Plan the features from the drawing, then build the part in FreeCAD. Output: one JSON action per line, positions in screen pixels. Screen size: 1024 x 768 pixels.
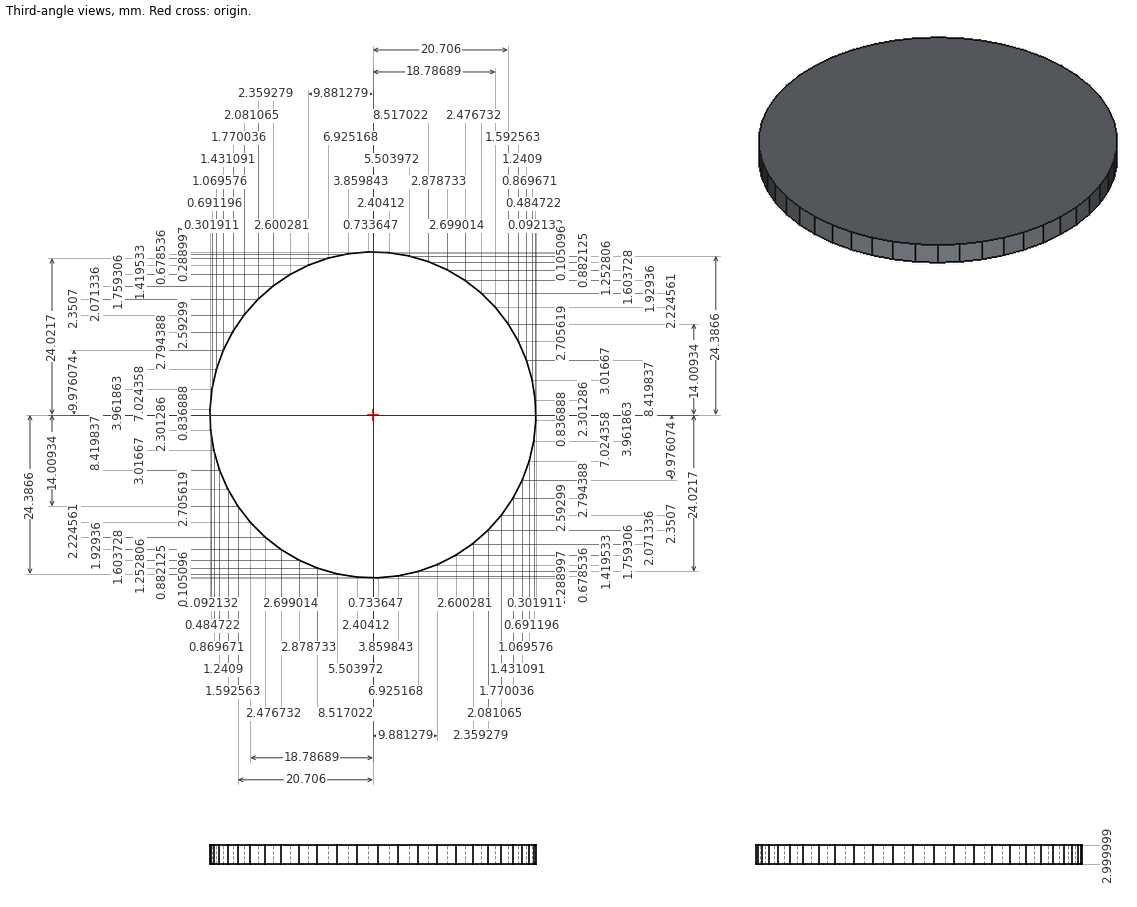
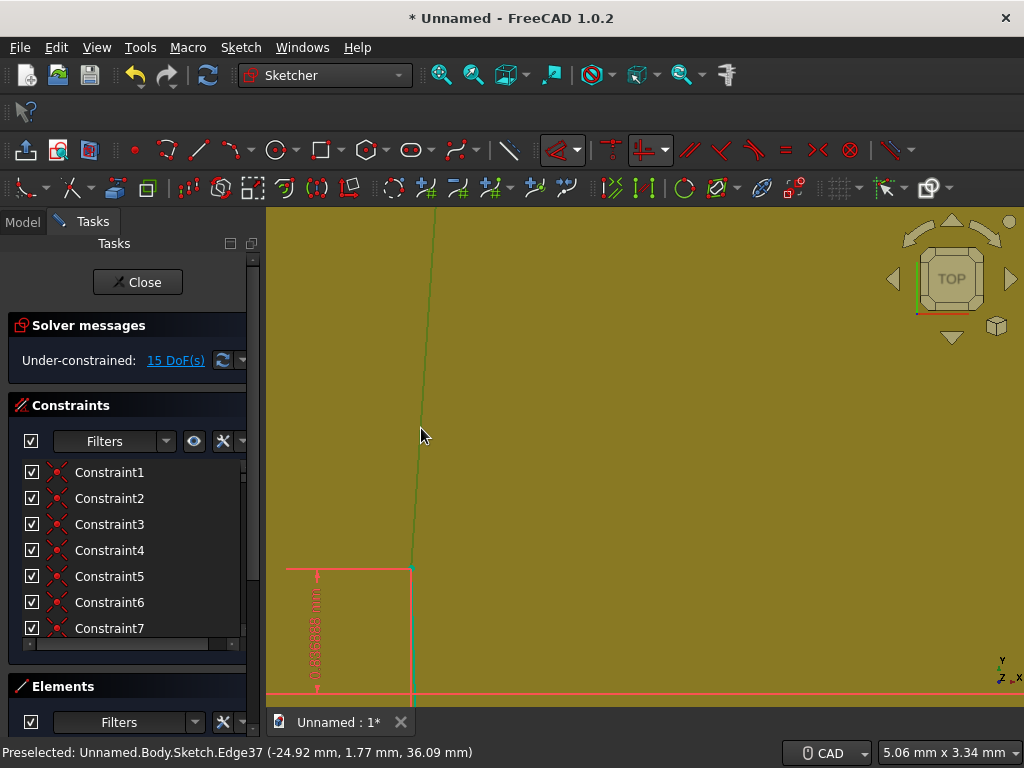
{"action": "left_click", "coordinate": [580, 150]}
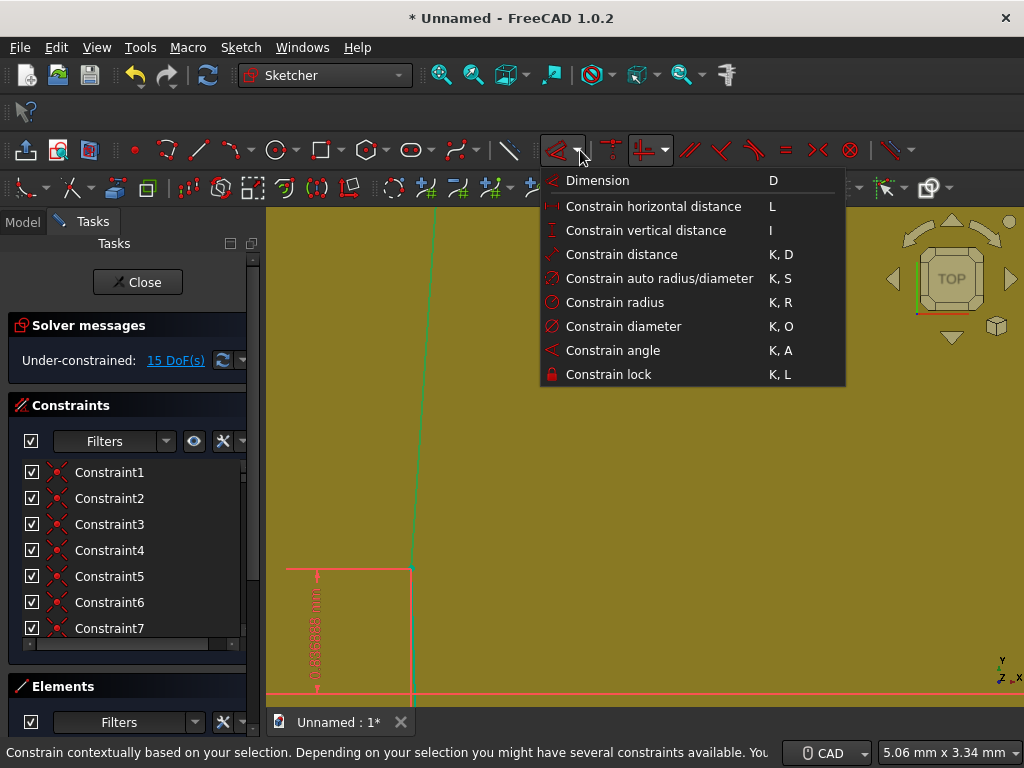
{"action": "left_click", "coordinate": [693, 206]}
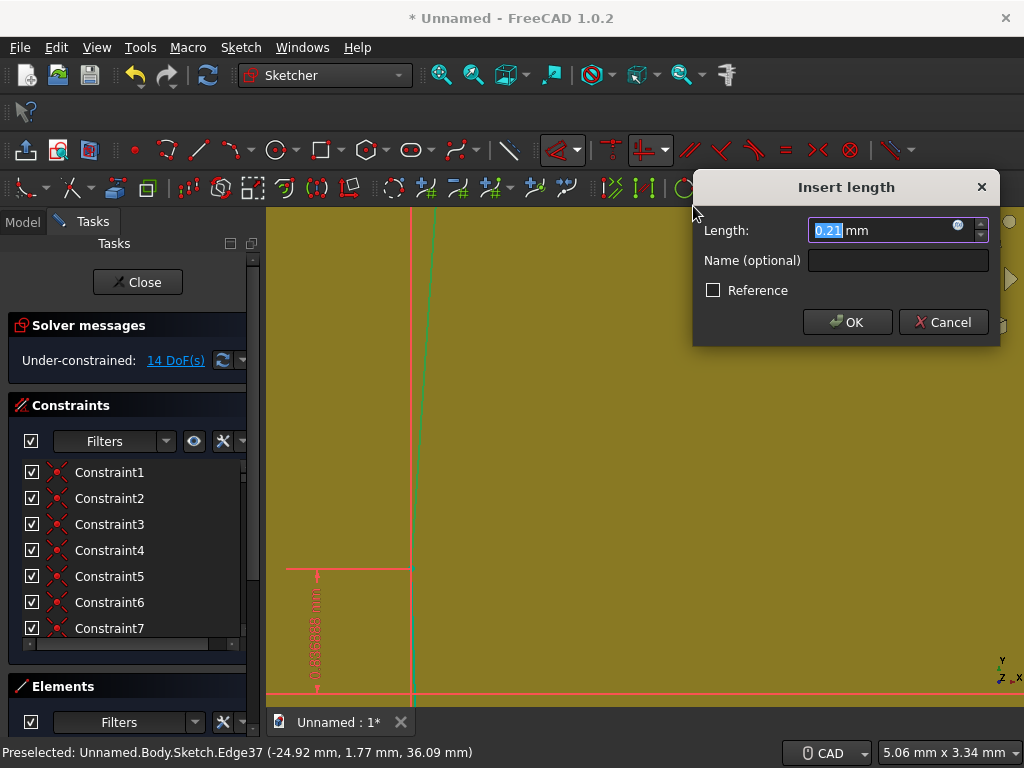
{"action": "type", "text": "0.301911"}
{"action": "key", "text": "Return"}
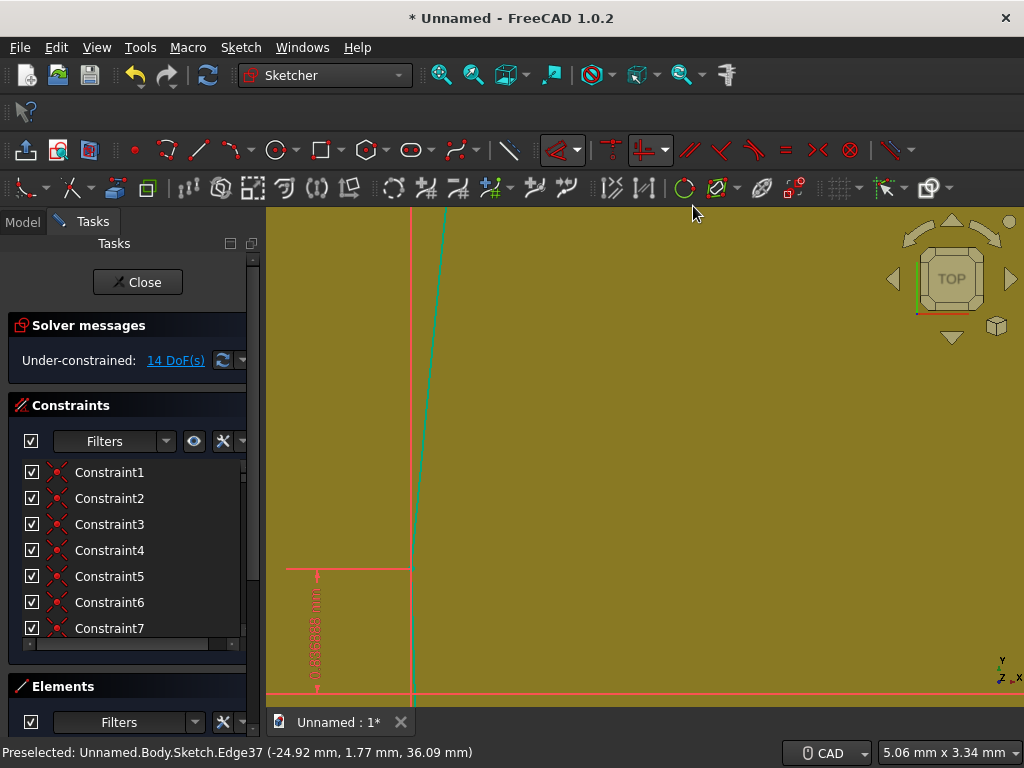
{"action": "scroll", "coordinate": [389, 445], "scroll_direction": "down", "scroll_amount": 15}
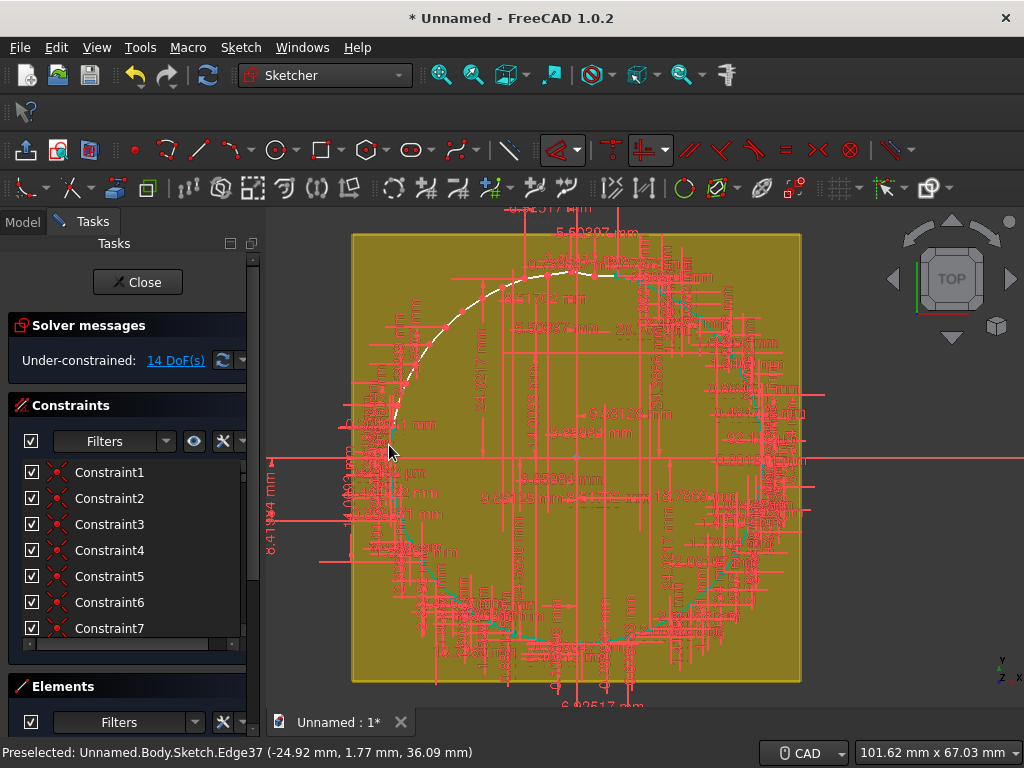
{"action": "scroll", "coordinate": [394, 421], "scroll_direction": "up", "scroll_amount": 11}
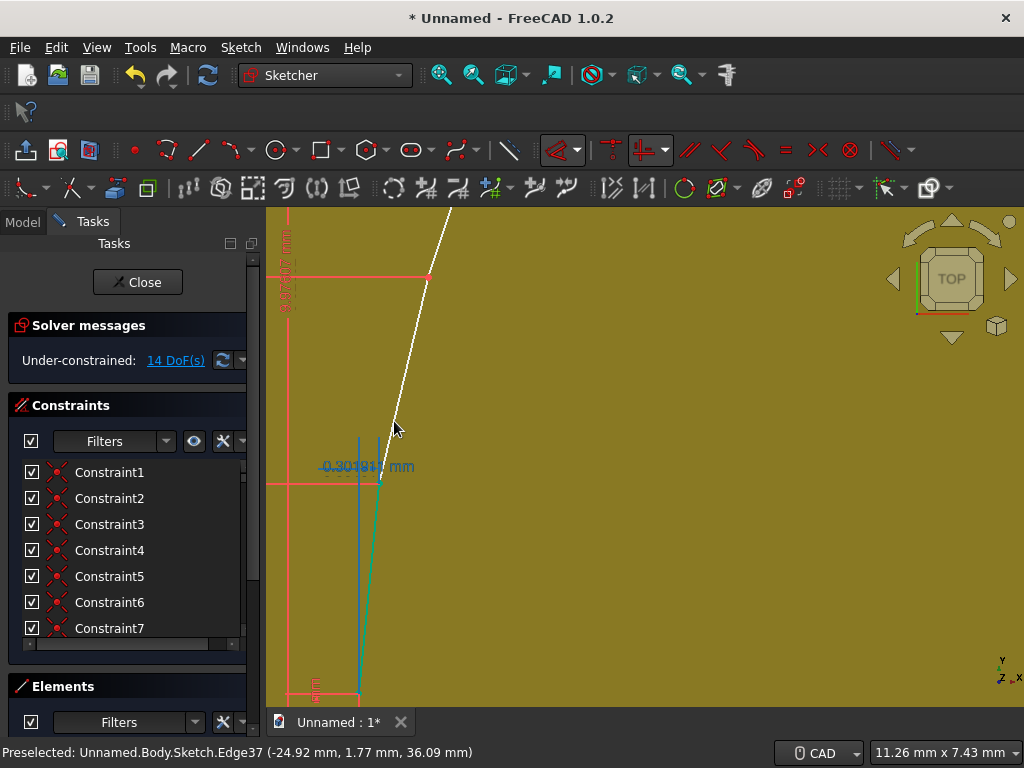
{"action": "left_click", "coordinate": [394, 422]}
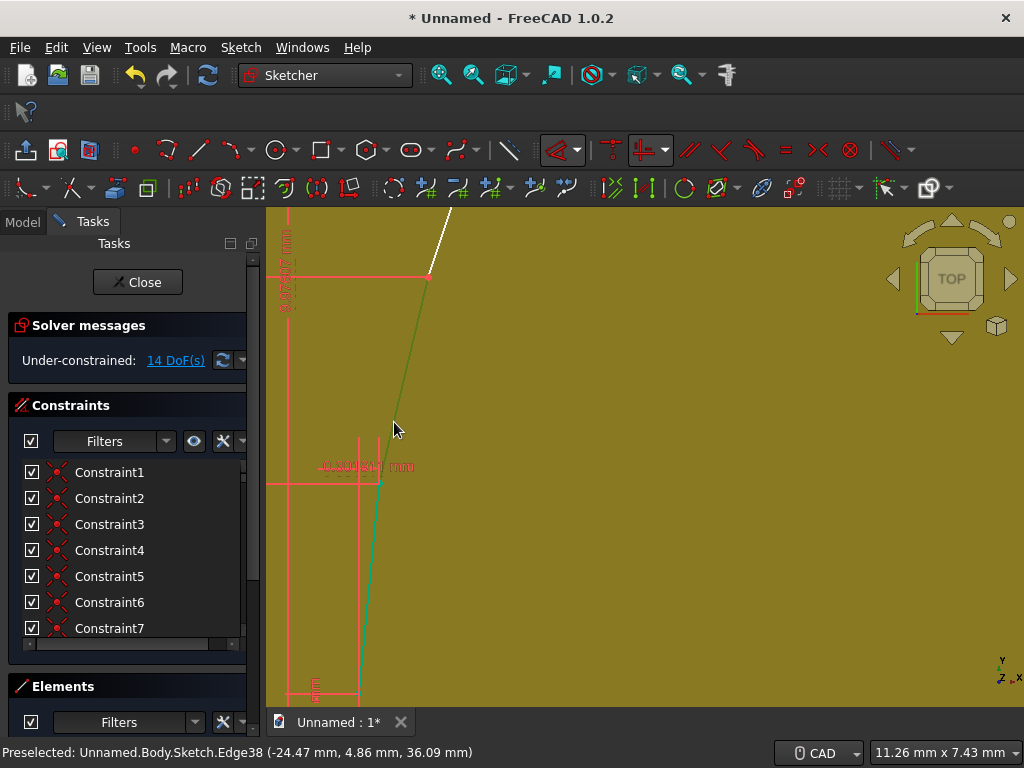
{"action": "left_click", "coordinate": [580, 150]}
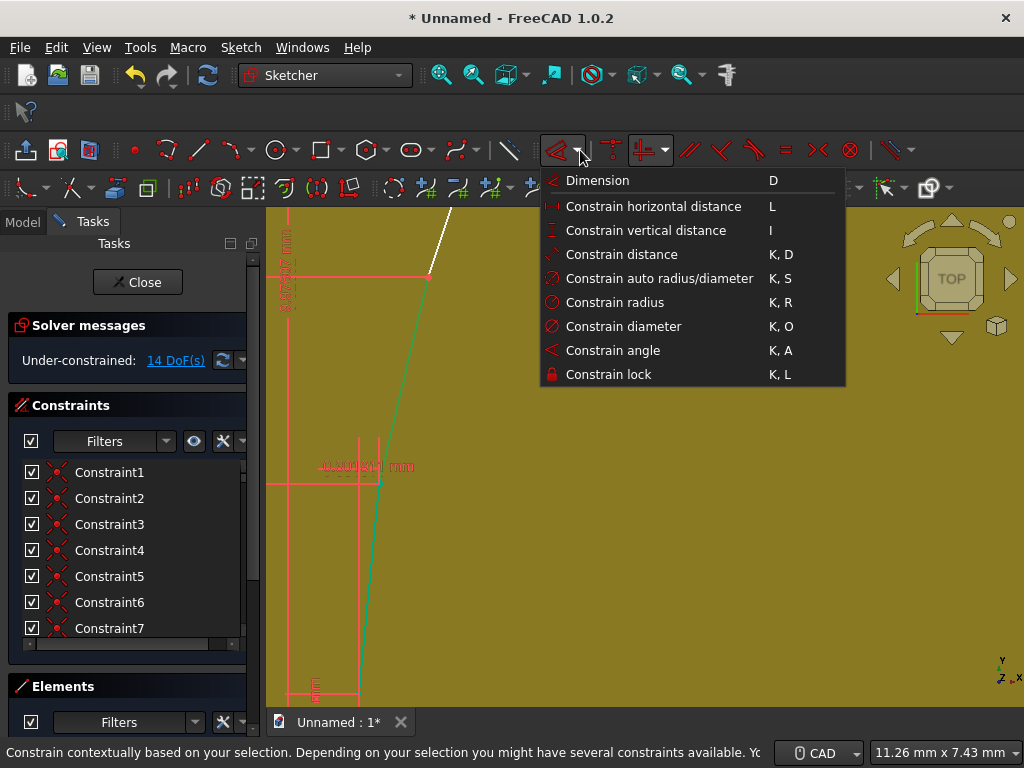
{"action": "left_click", "coordinate": [693, 206]}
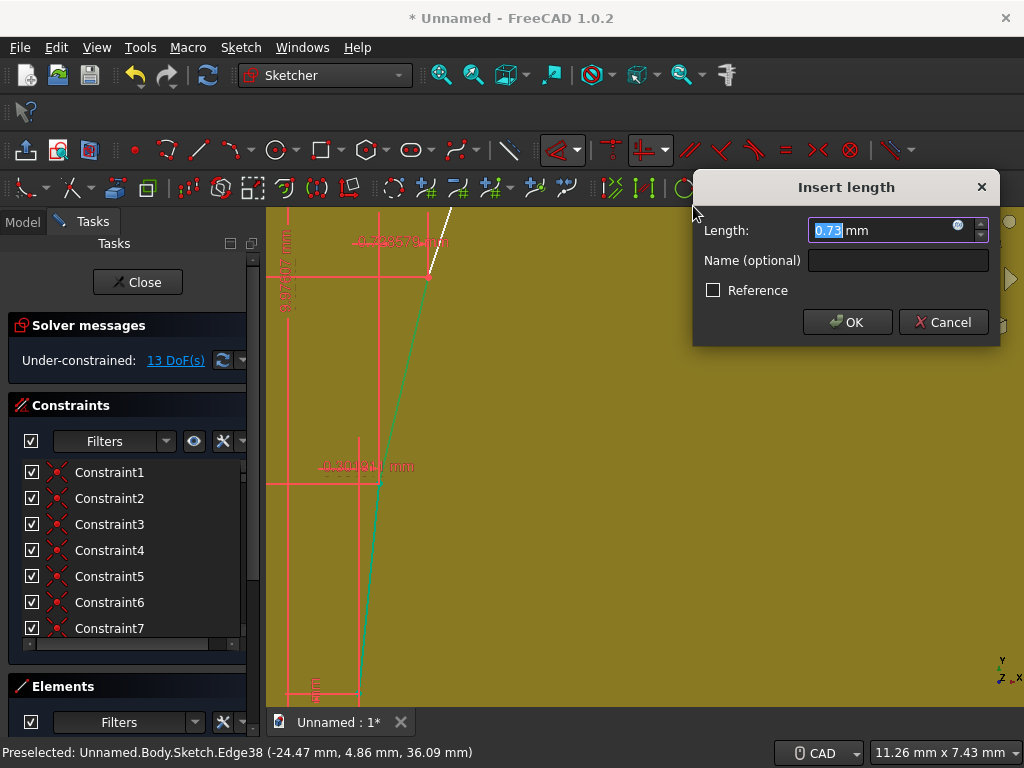
{"action": "type", "text": "0.691196"}
{"action": "key", "text": "Return"}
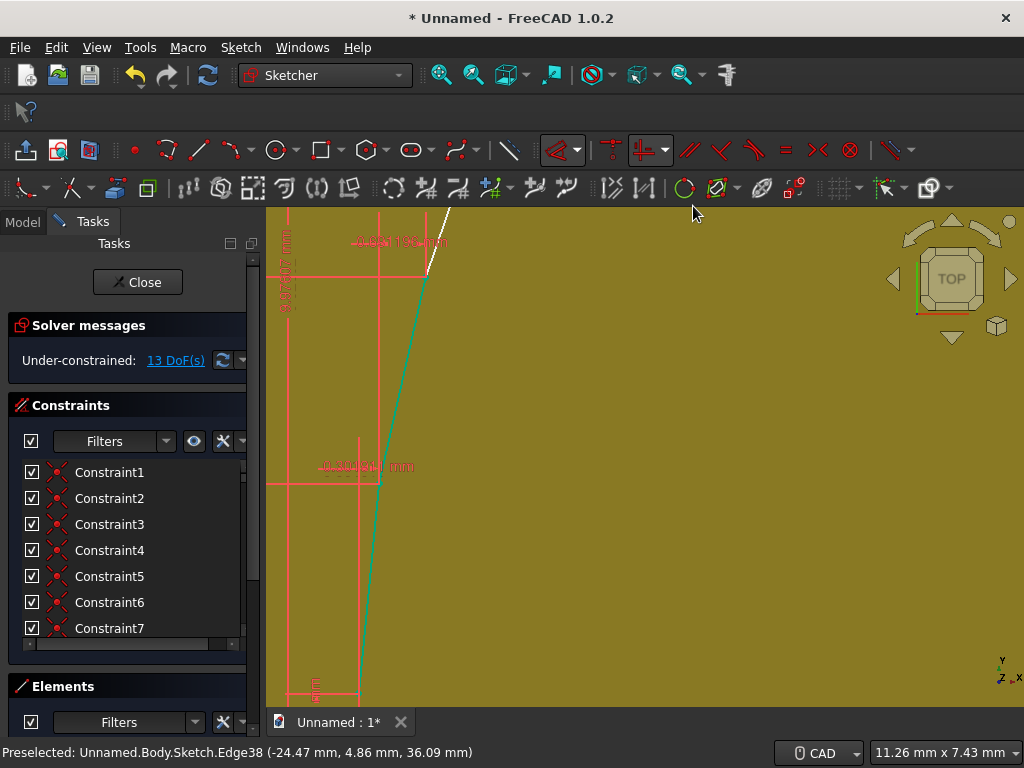
{"action": "scroll", "coordinate": [439, 238], "scroll_direction": "up", "scroll_amount": 4}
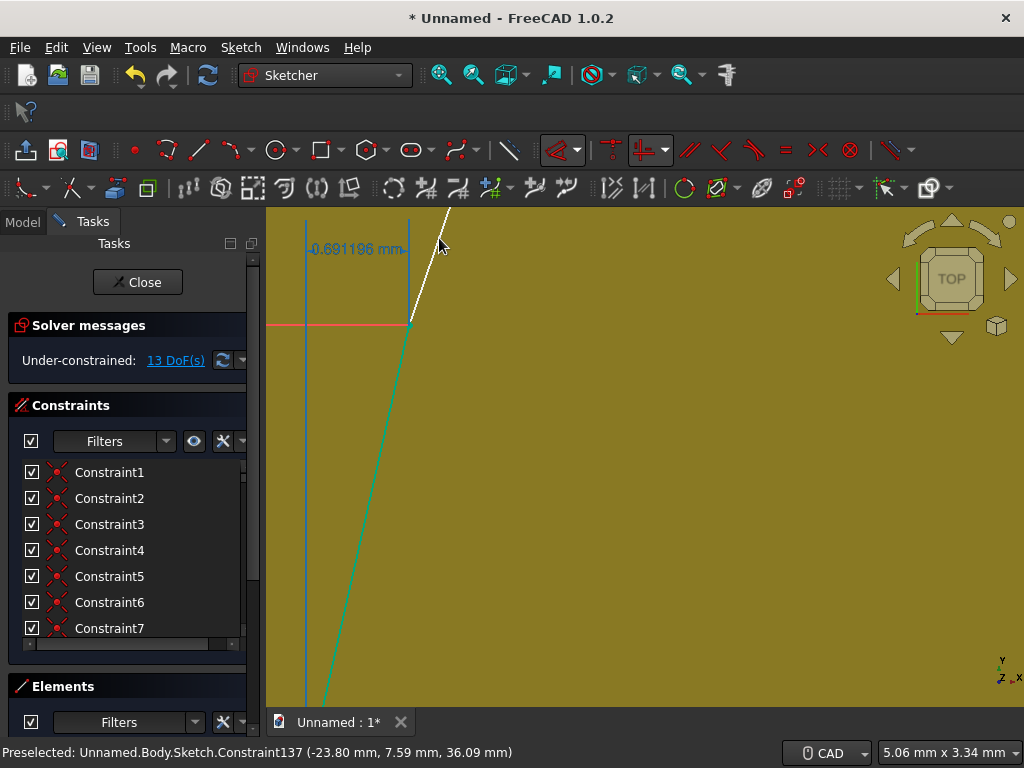
{"action": "left_click", "coordinate": [440, 237]}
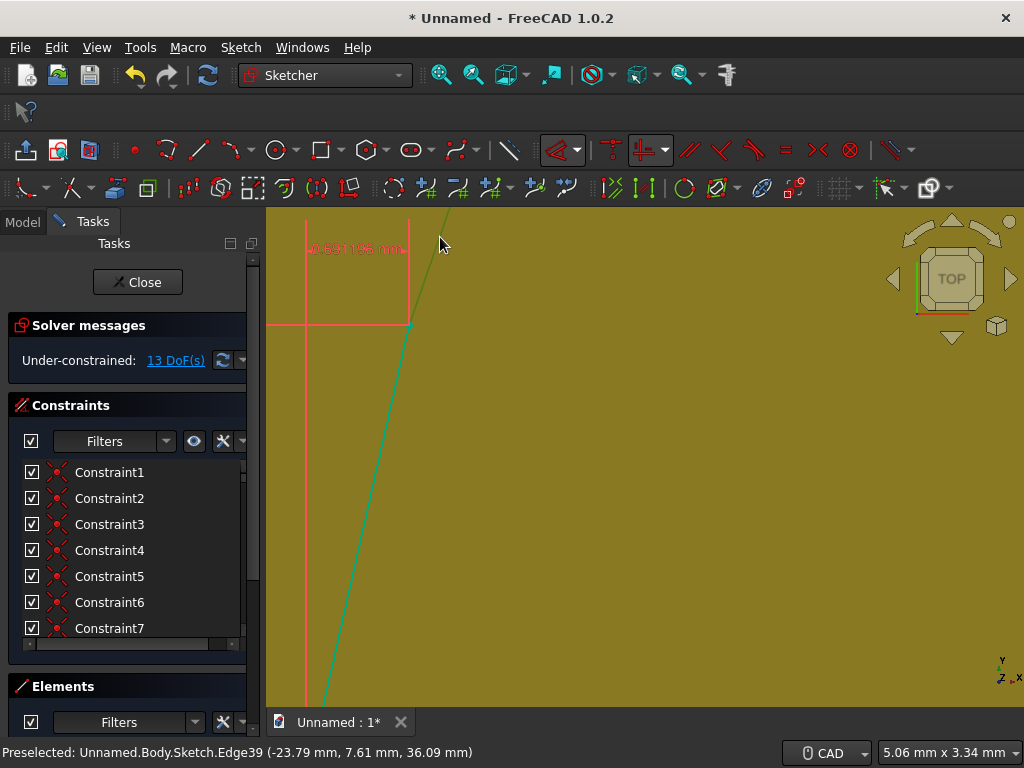
{"action": "key", "text": "l"}